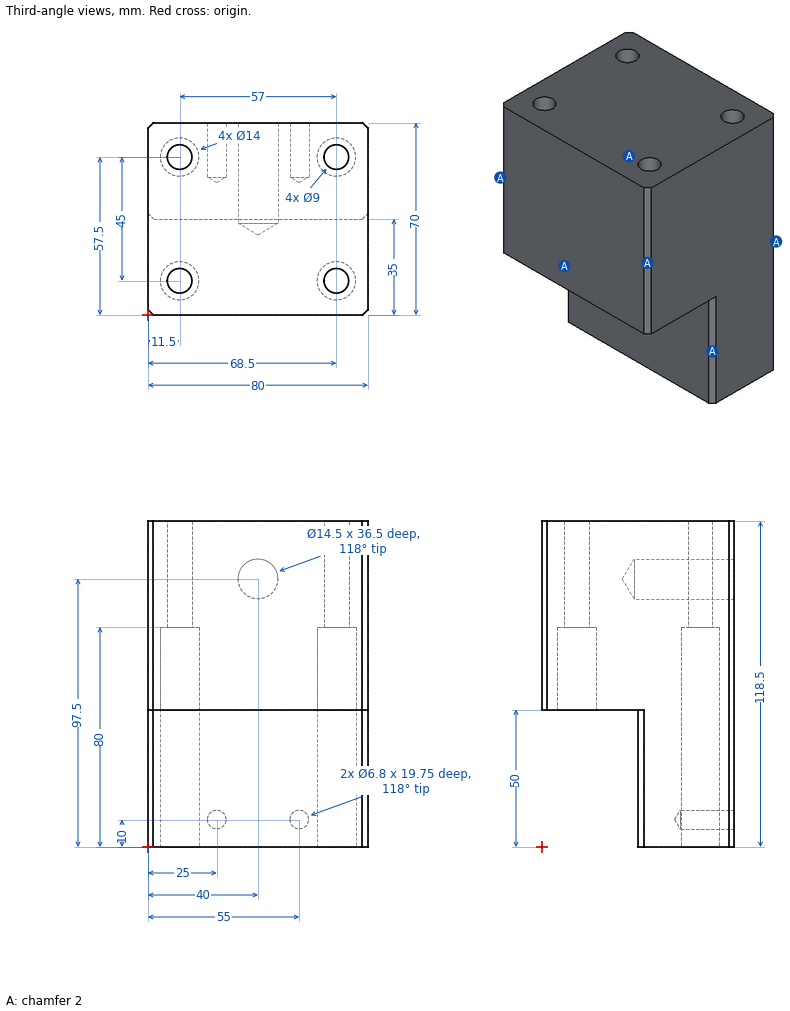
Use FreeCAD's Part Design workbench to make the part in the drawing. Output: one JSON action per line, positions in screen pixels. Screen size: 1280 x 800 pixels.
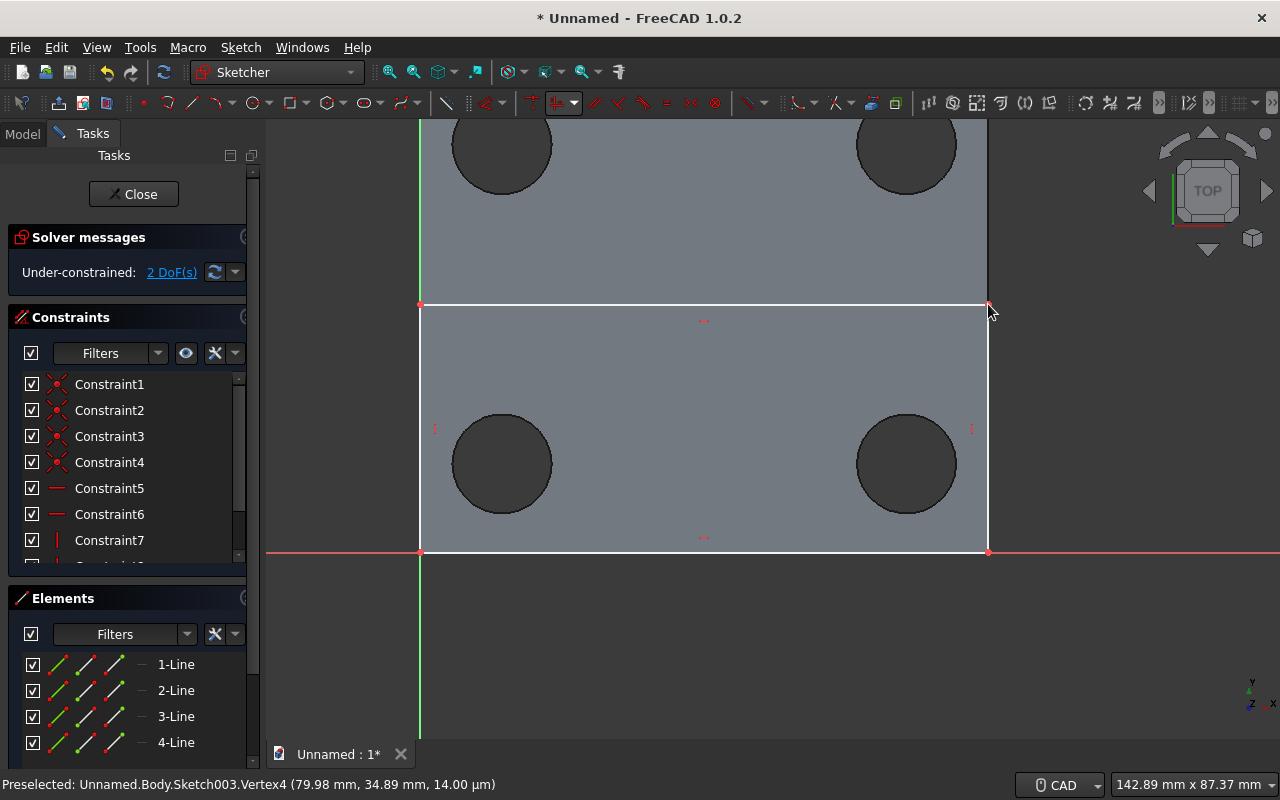
{"action": "key", "text": "d"}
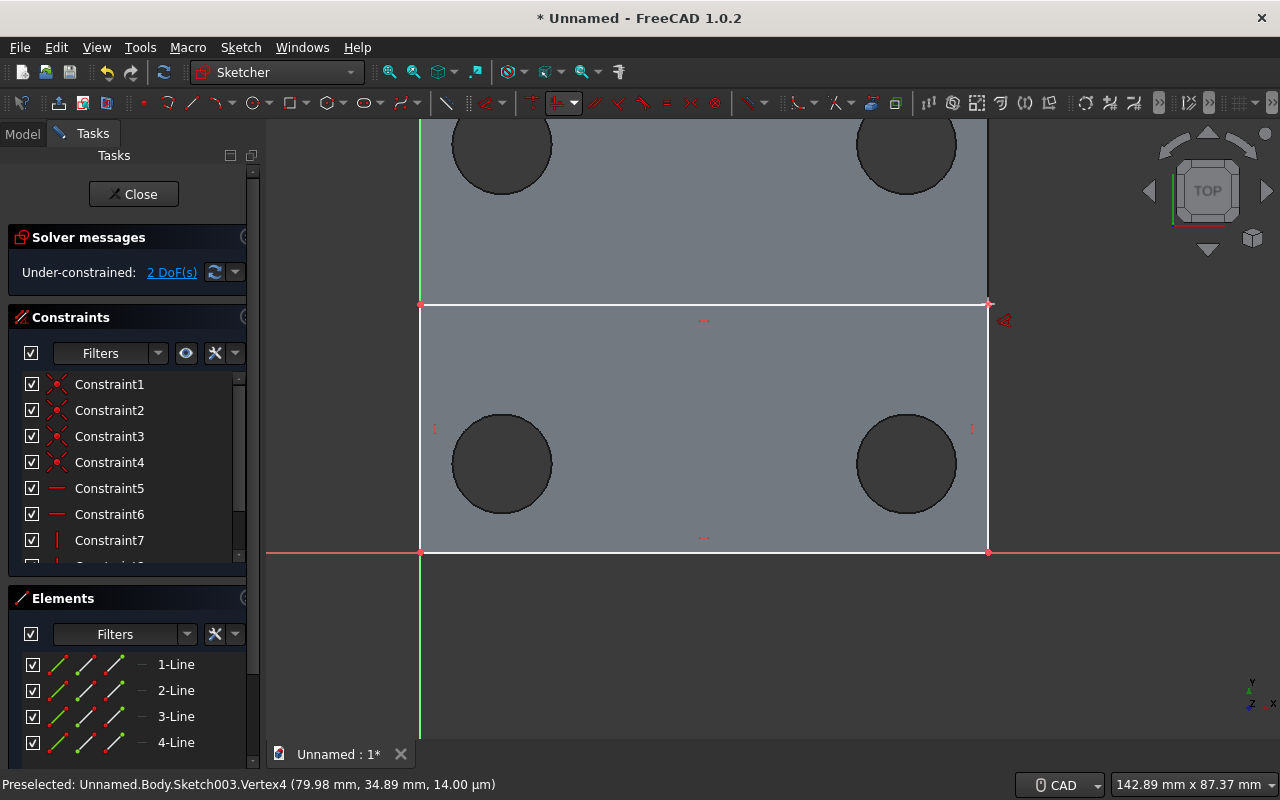
{"action": "left_click", "coordinate": [591, 553]}
{"action": "left_click", "coordinate": [704, 587]}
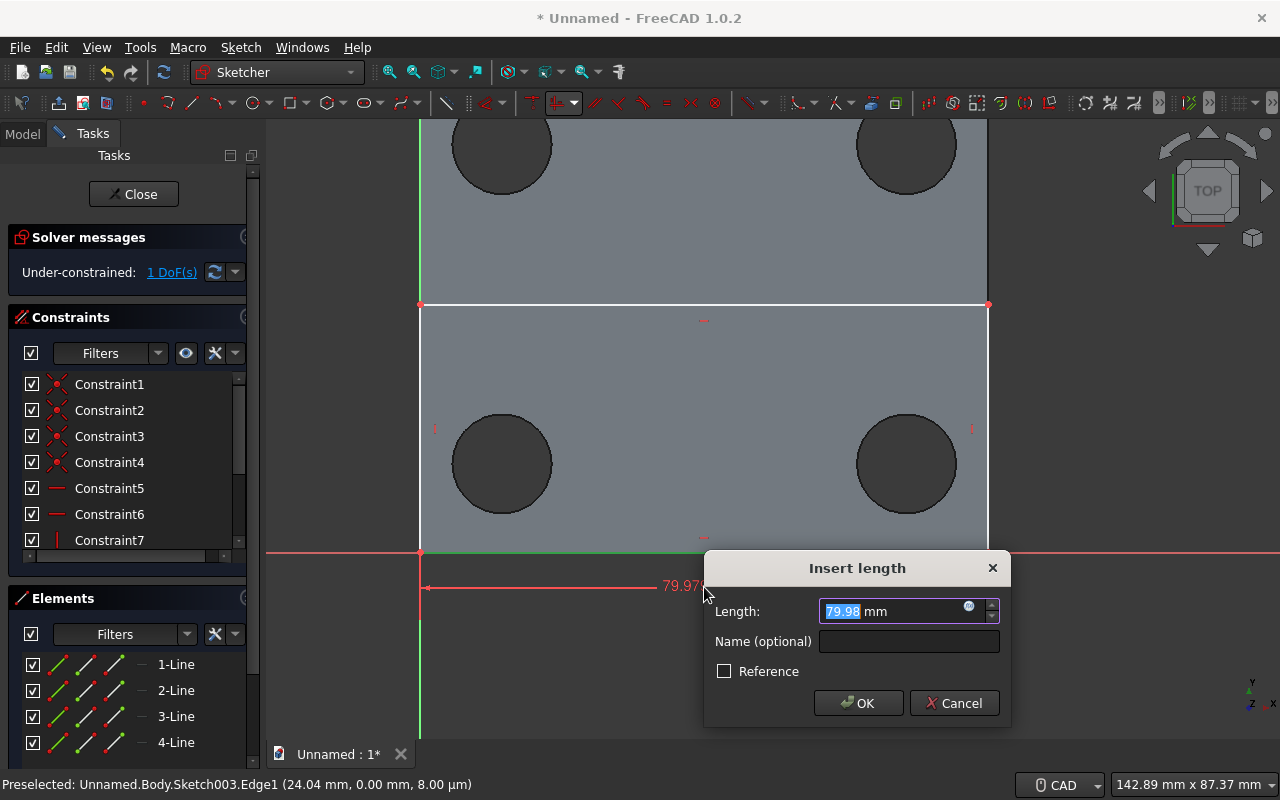
{"action": "type", "text": "80"}
{"action": "key", "text": "Return"}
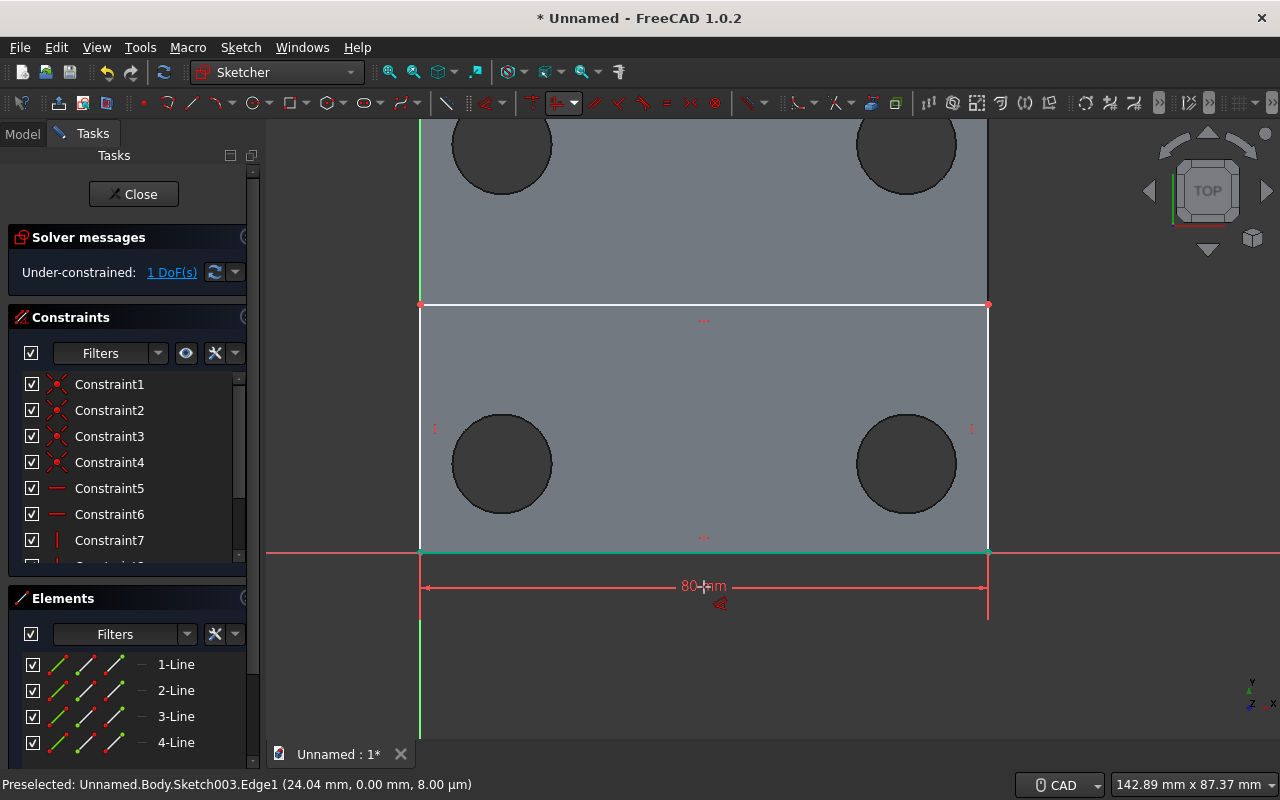
{"action": "left_click", "coordinate": [988, 478]}
{"action": "left_click", "coordinate": [1022, 429]}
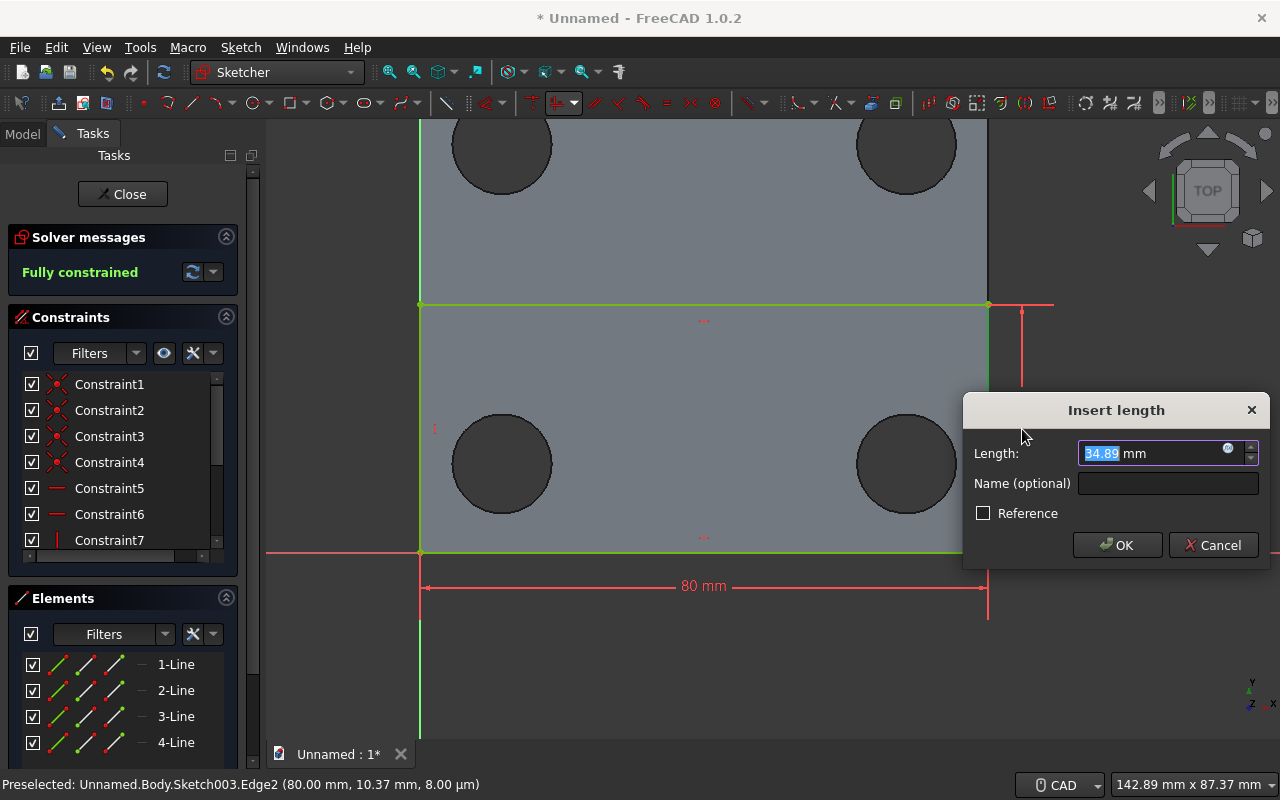
{"action": "type", "text": "35"}
{"action": "key", "text": "Return"}
{"action": "key", "text": "Escape"}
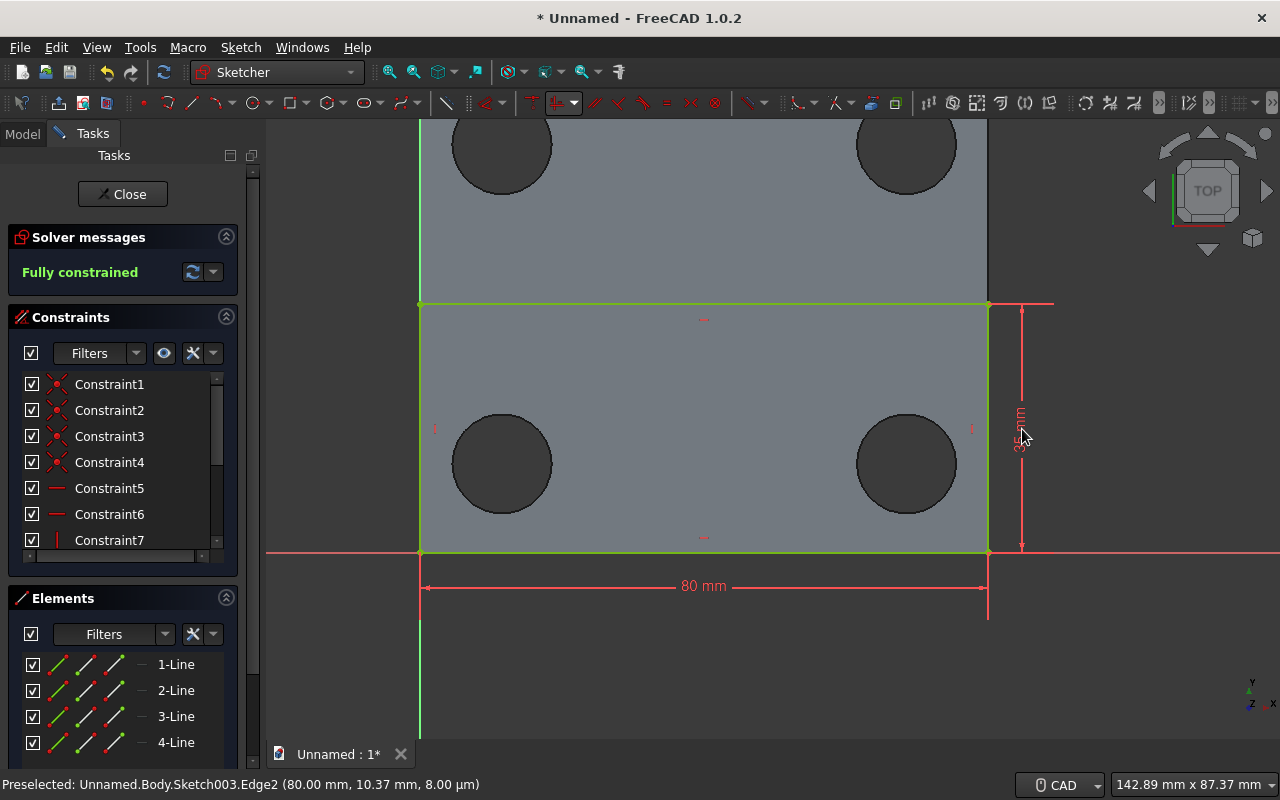
{"action": "left_click", "coordinate": [123, 194]}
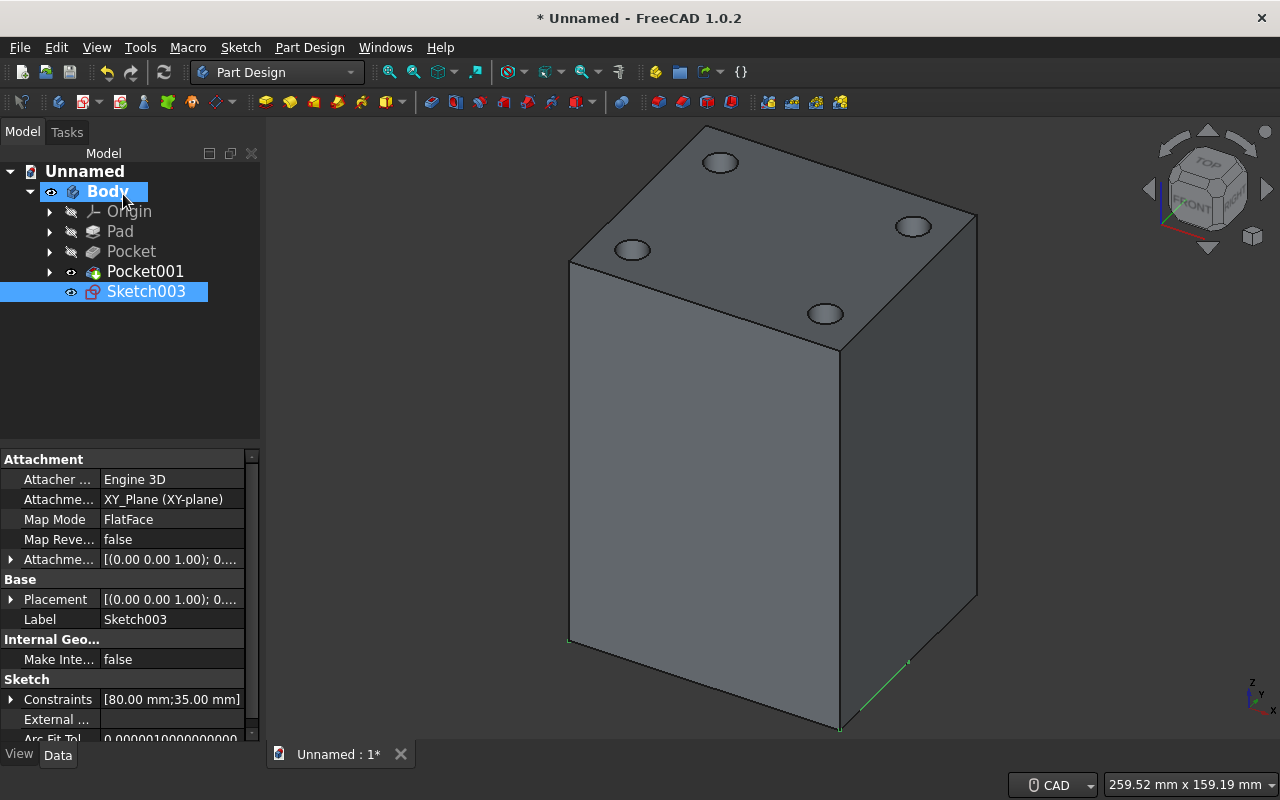
{"action": "left_click", "coordinate": [432, 102]}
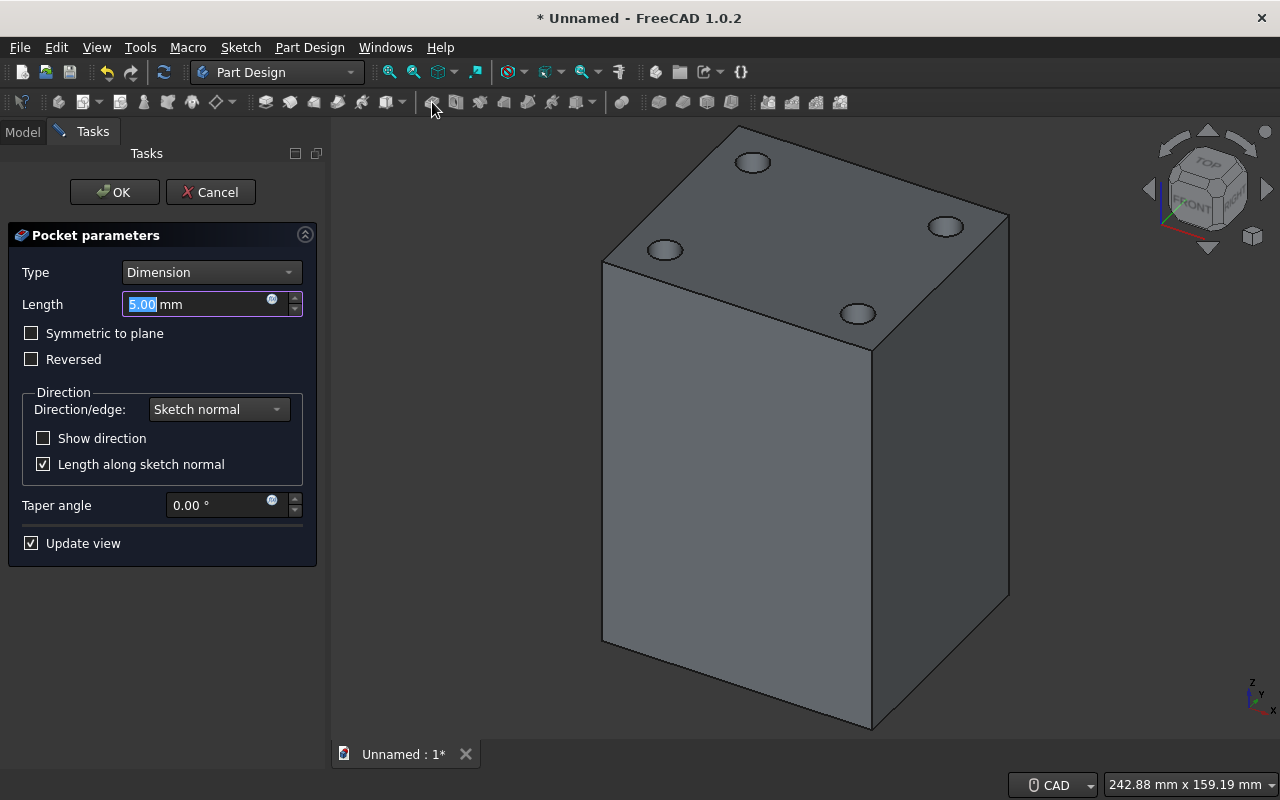
{"action": "type", "text": "50"}
{"action": "key", "text": "Tab"}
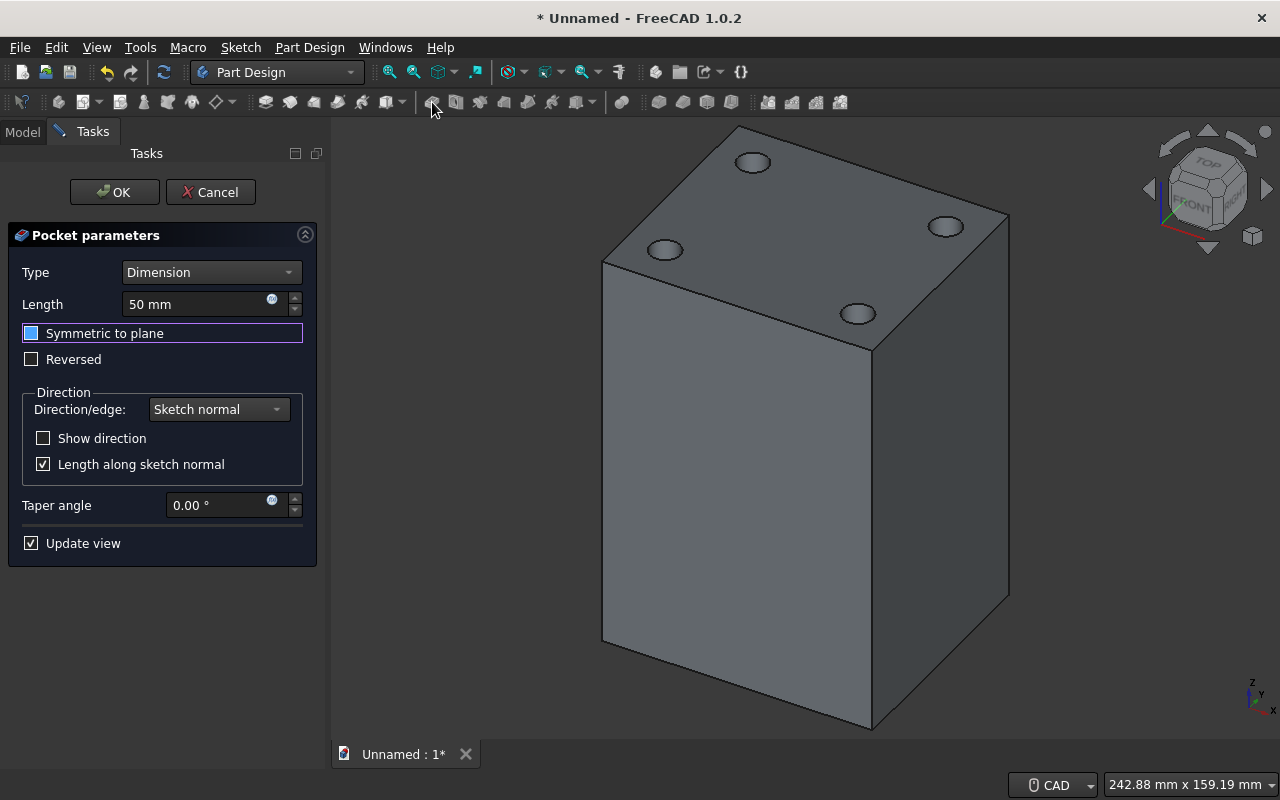
{"action": "left_click", "coordinate": [30, 359]}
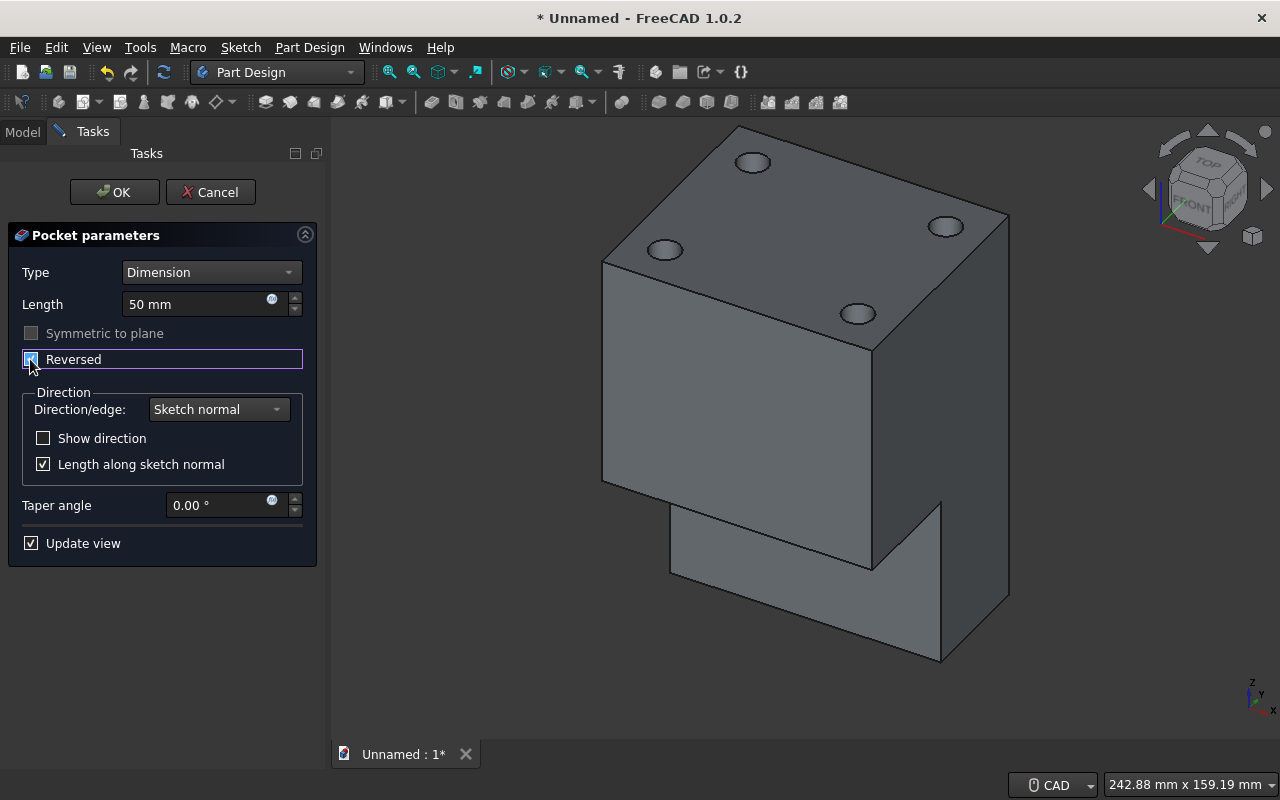
{"action": "left_click", "coordinate": [115, 192]}